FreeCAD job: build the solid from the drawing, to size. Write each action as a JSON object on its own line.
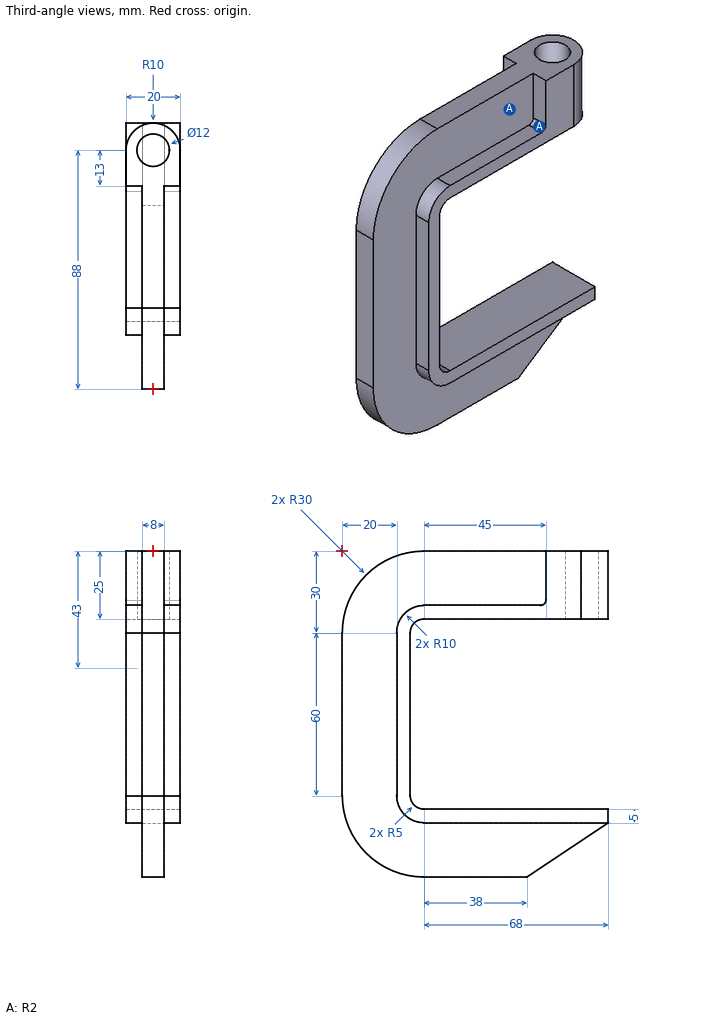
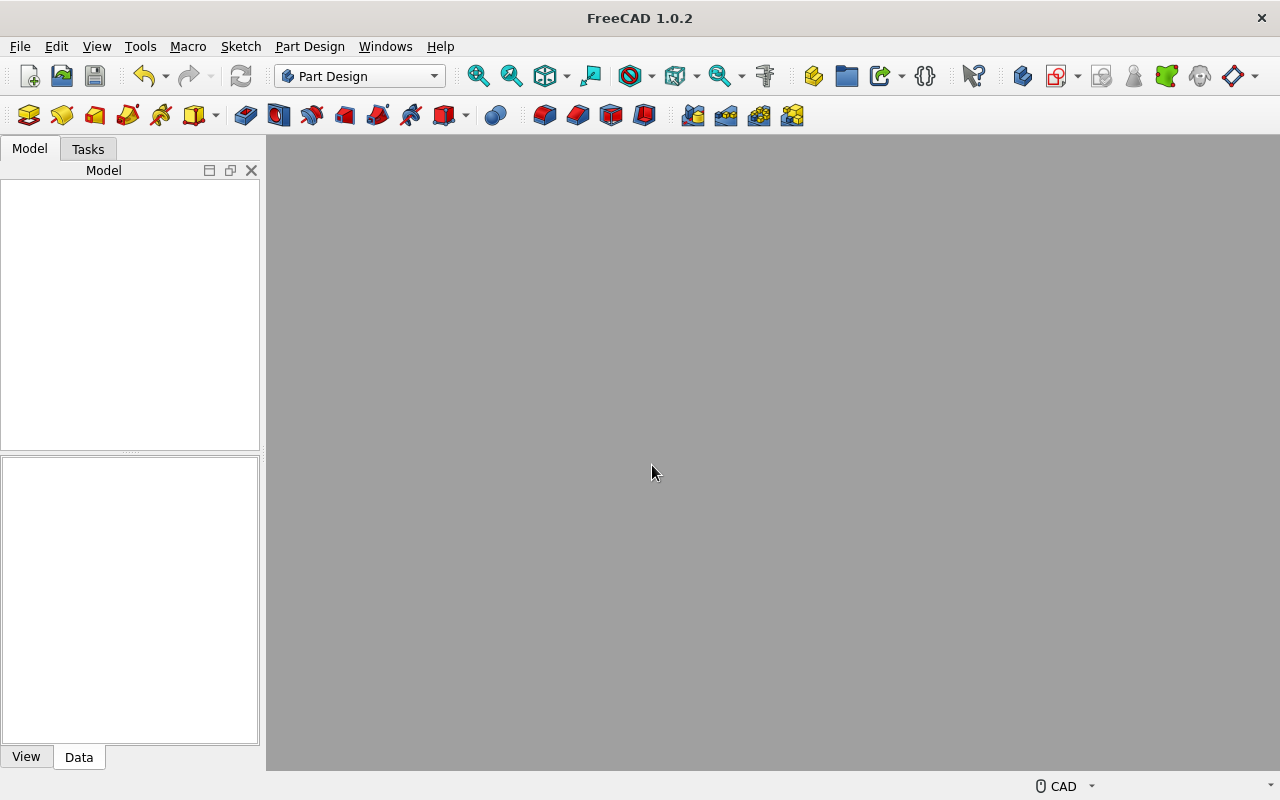
{"action": "key", "text": "ctrl+n"}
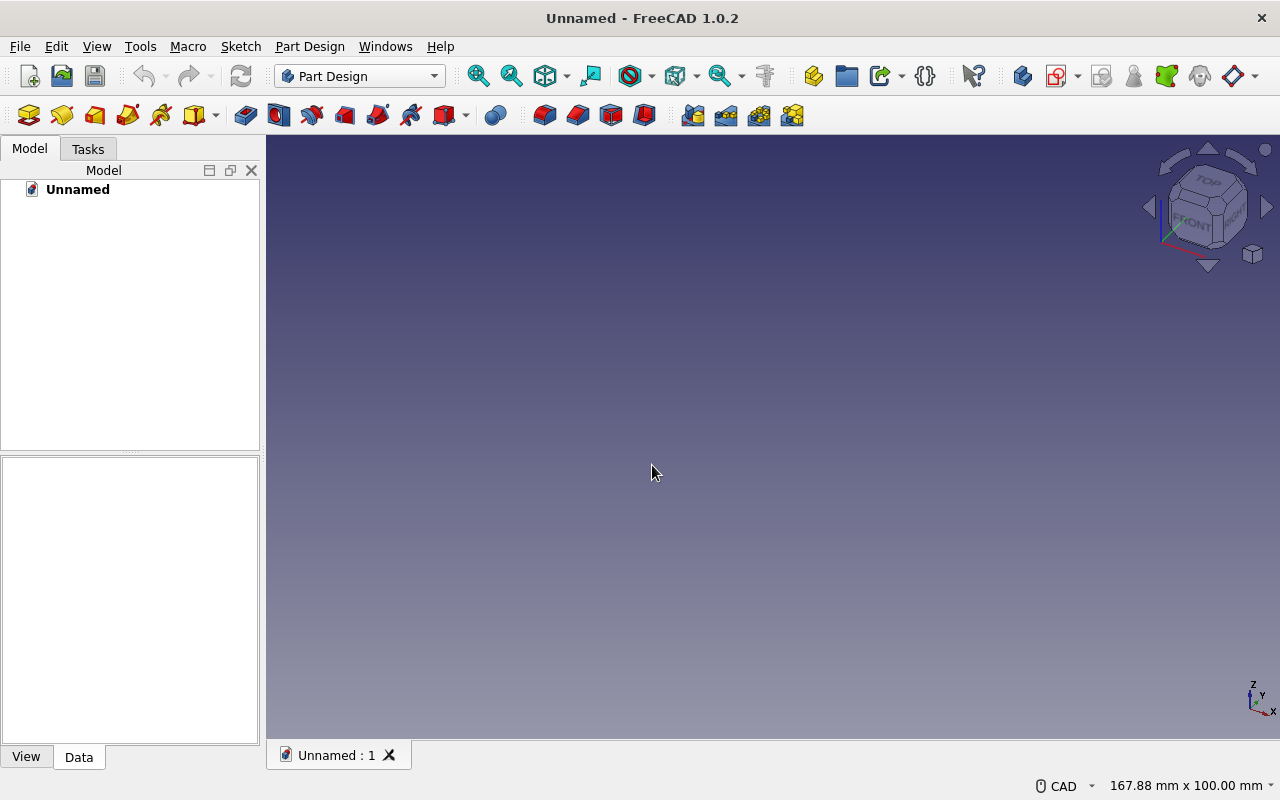
{"action": "left_click", "coordinate": [1056, 76]}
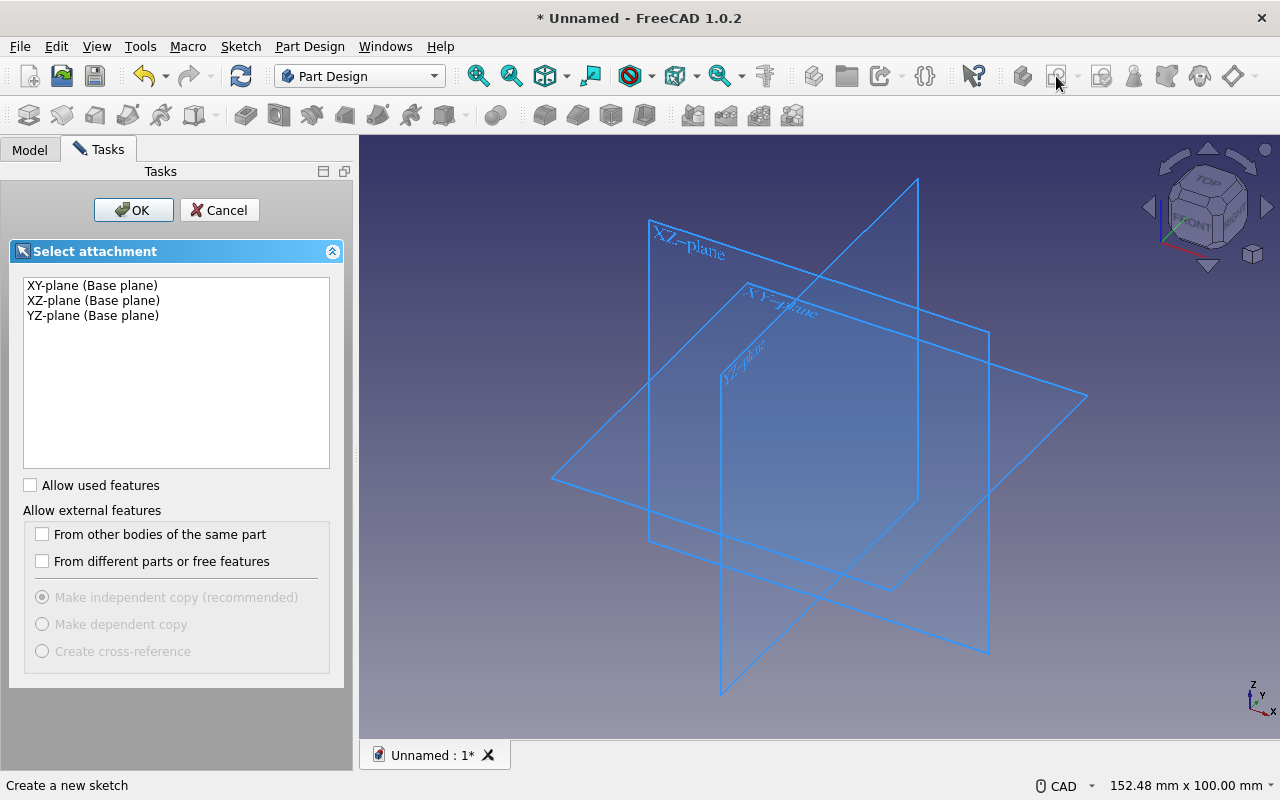
{"action": "left_click", "coordinate": [84, 316]}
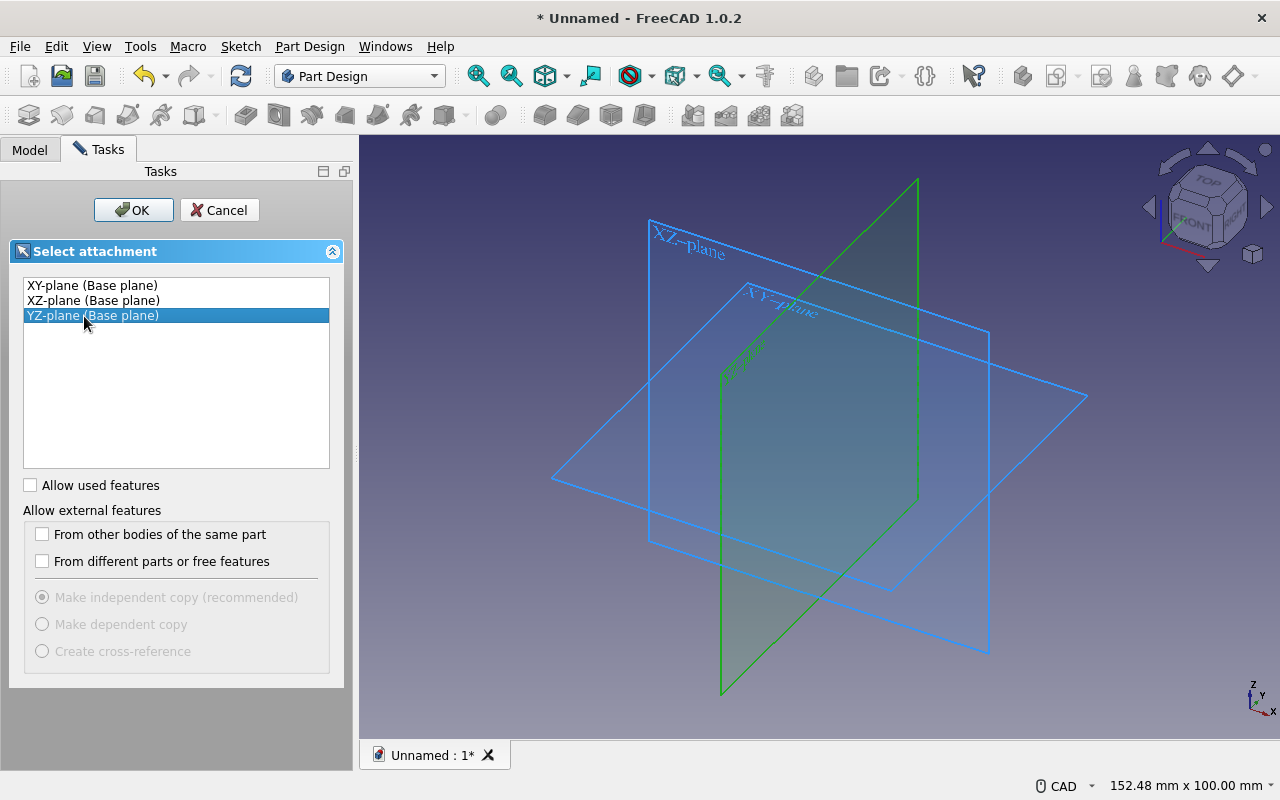
{"action": "left_click", "coordinate": [134, 210]}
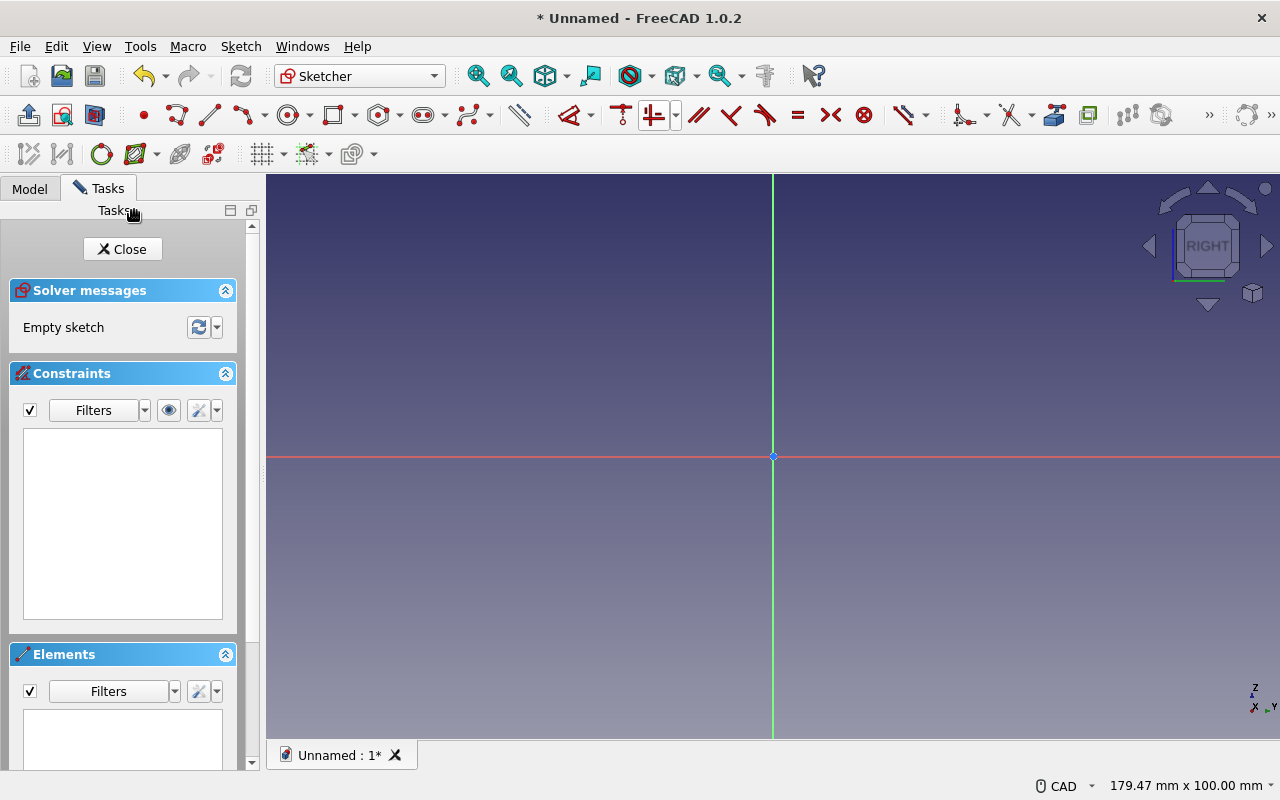
{"action": "scroll", "coordinate": [423, 202], "scroll_direction": "down", "scroll_amount": 4}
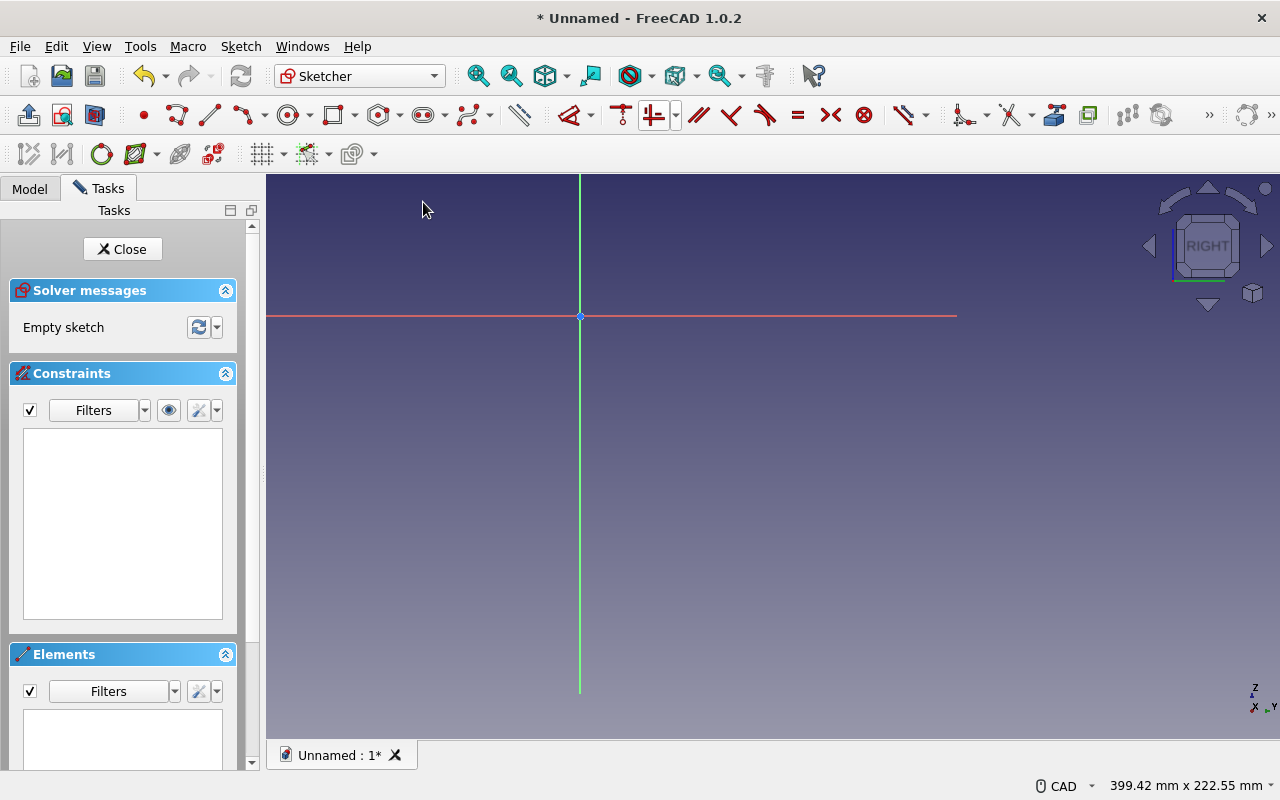
{"action": "left_click", "coordinate": [210, 116]}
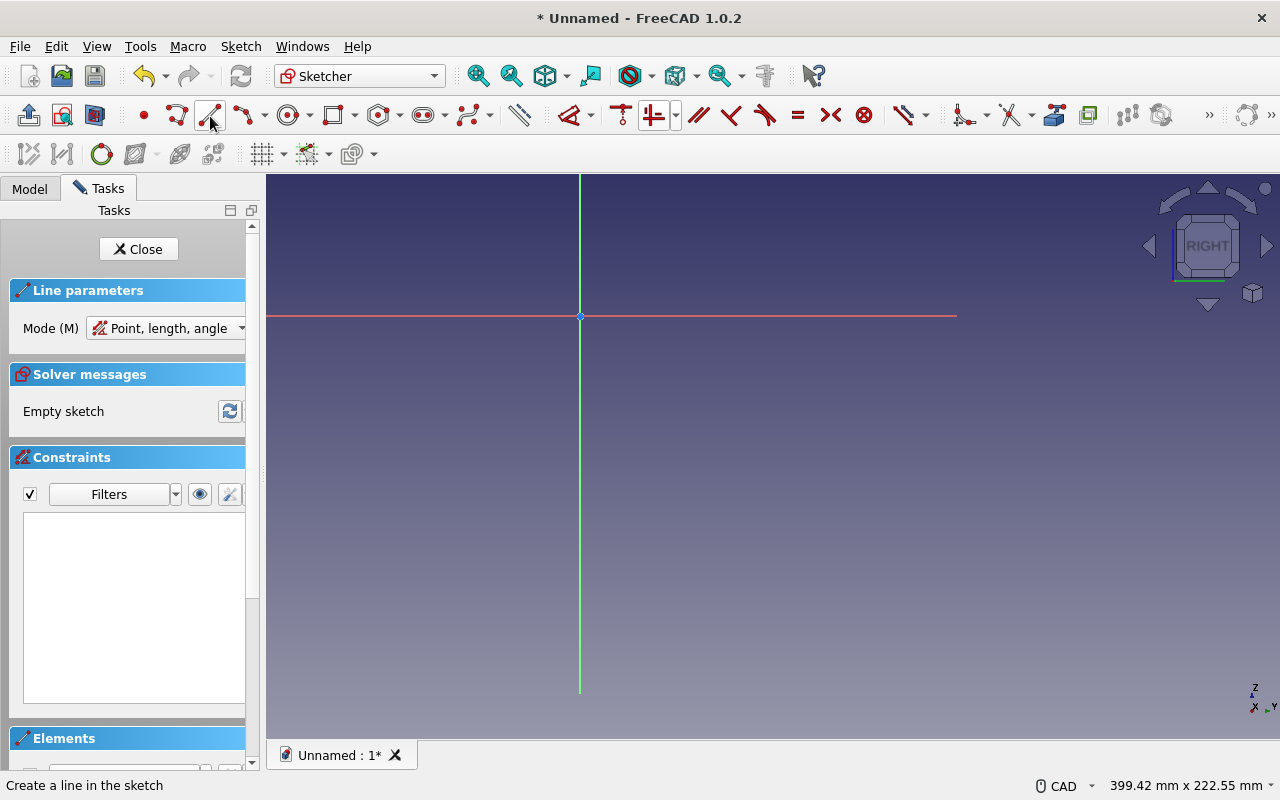
{"action": "left_click", "coordinate": [580, 393]}
{"action": "left_click", "coordinate": [589, 545]}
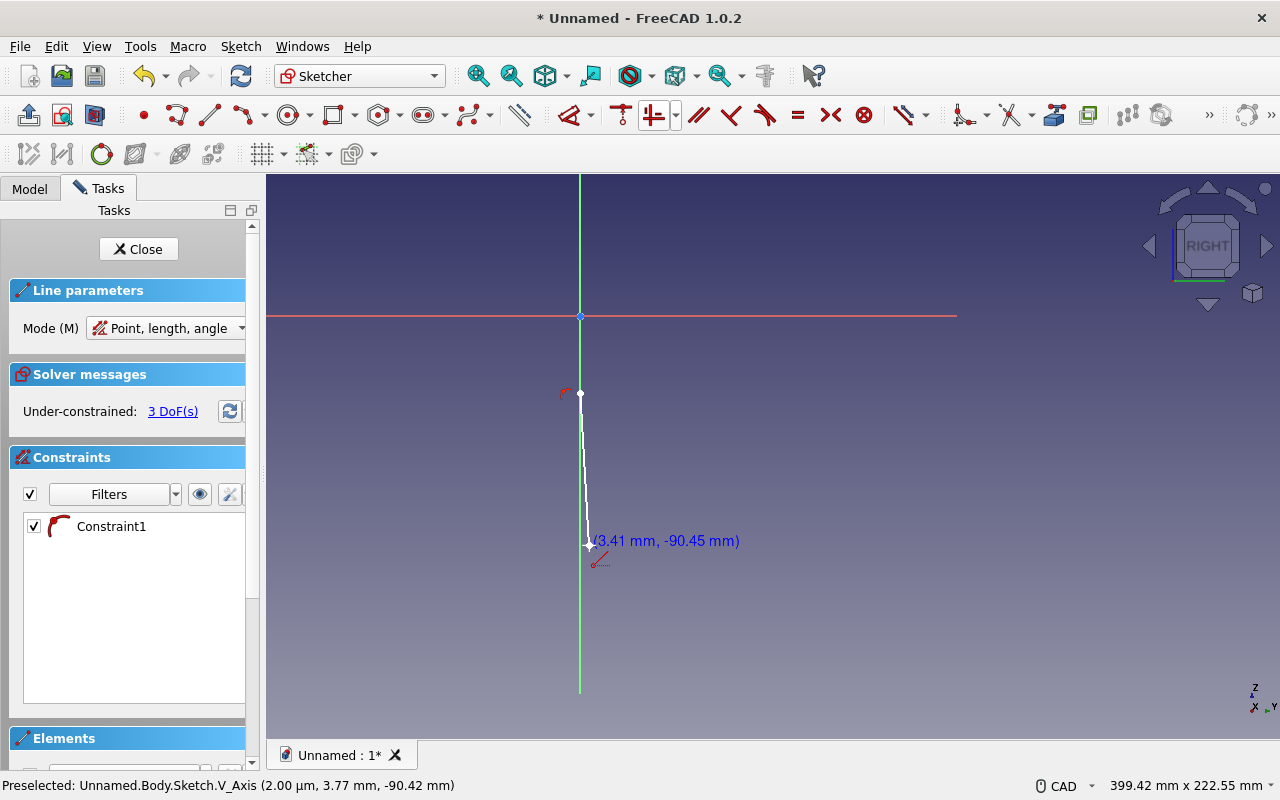
{"action": "left_click", "coordinate": [177, 116]}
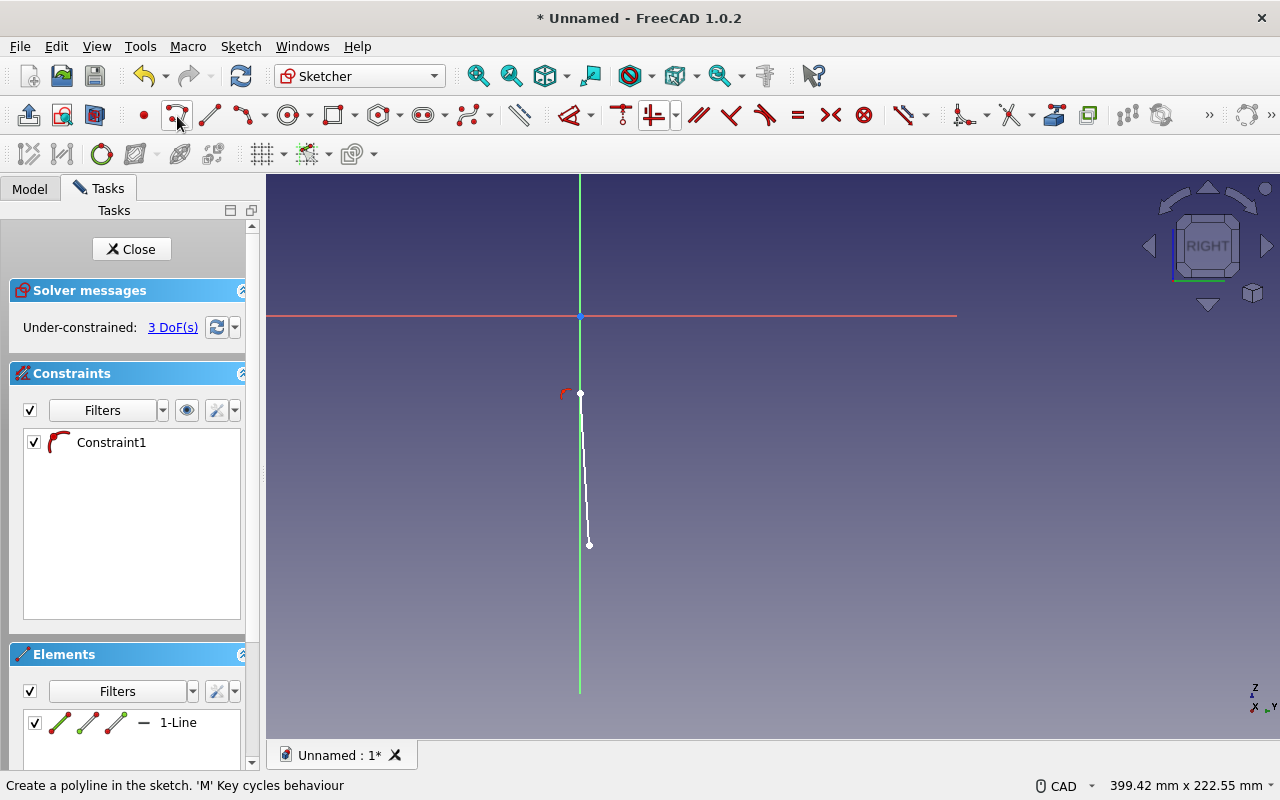
{"action": "left_click", "coordinate": [657, 621]}
{"action": "left_click", "coordinate": [753, 621]}
{"action": "left_click", "coordinate": [829, 570]}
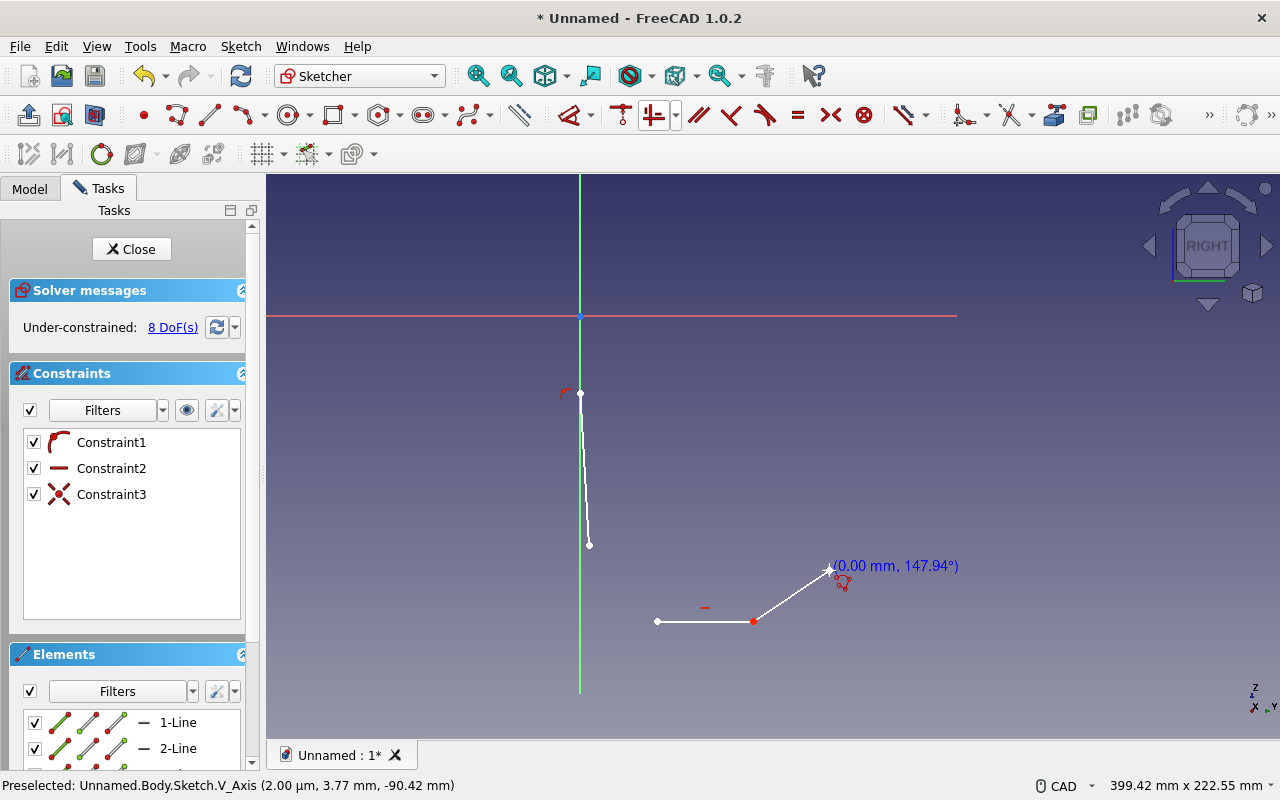
{"action": "scroll", "coordinate": [829, 558], "scroll_direction": "up", "scroll_amount": 2}